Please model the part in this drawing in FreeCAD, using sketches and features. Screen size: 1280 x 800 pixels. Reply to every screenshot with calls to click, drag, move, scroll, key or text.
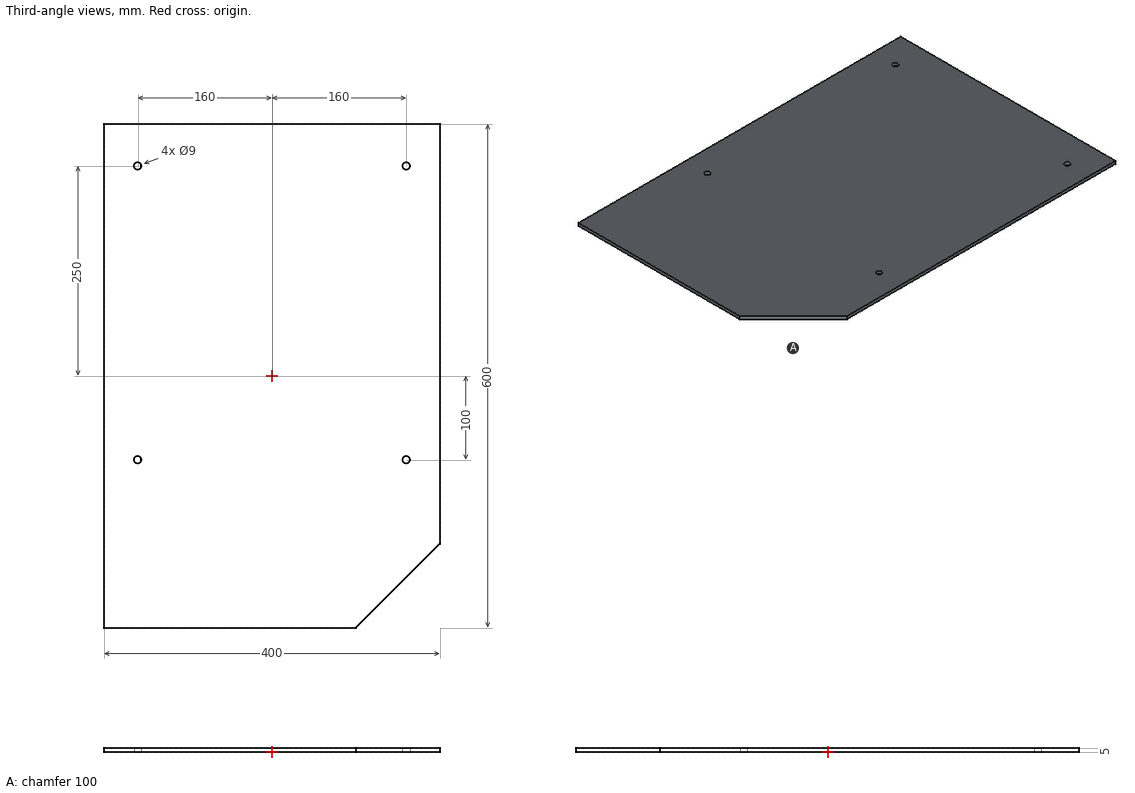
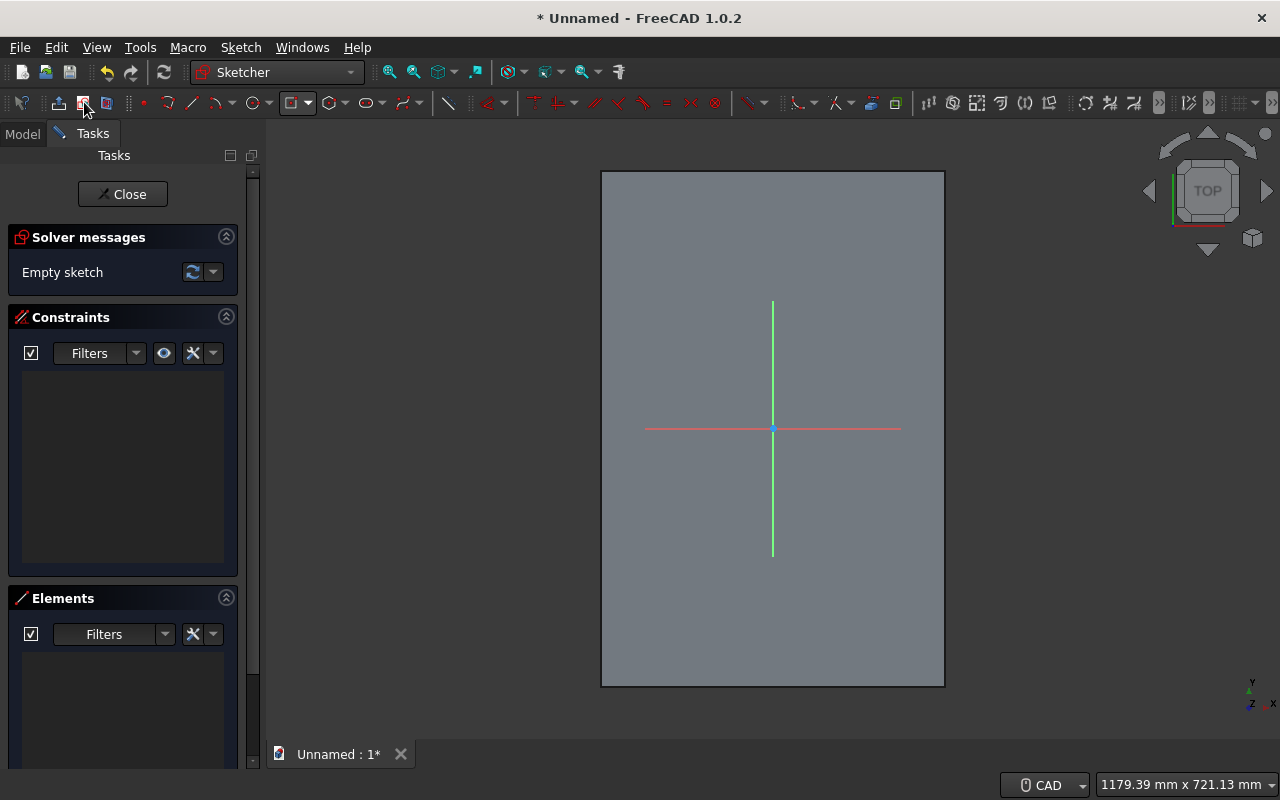
click(254, 104)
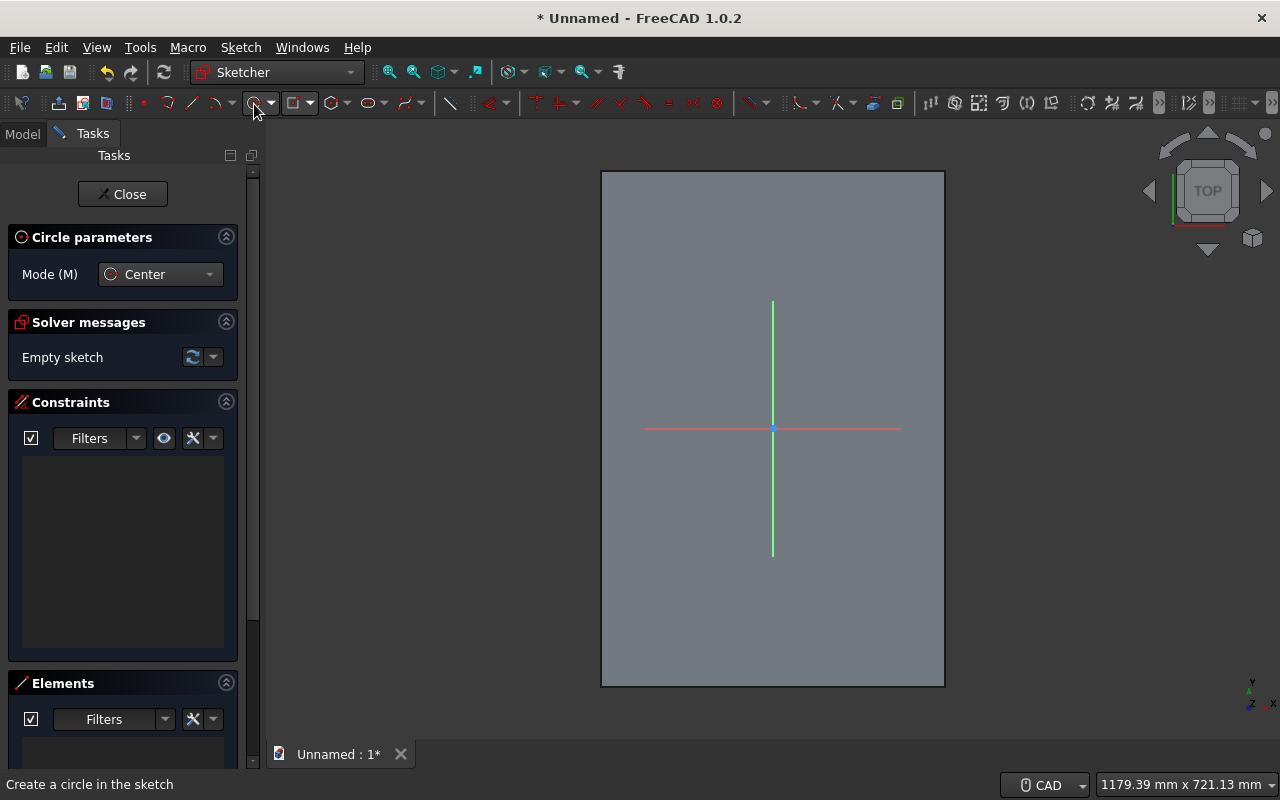
scroll(635, 214, up, 9)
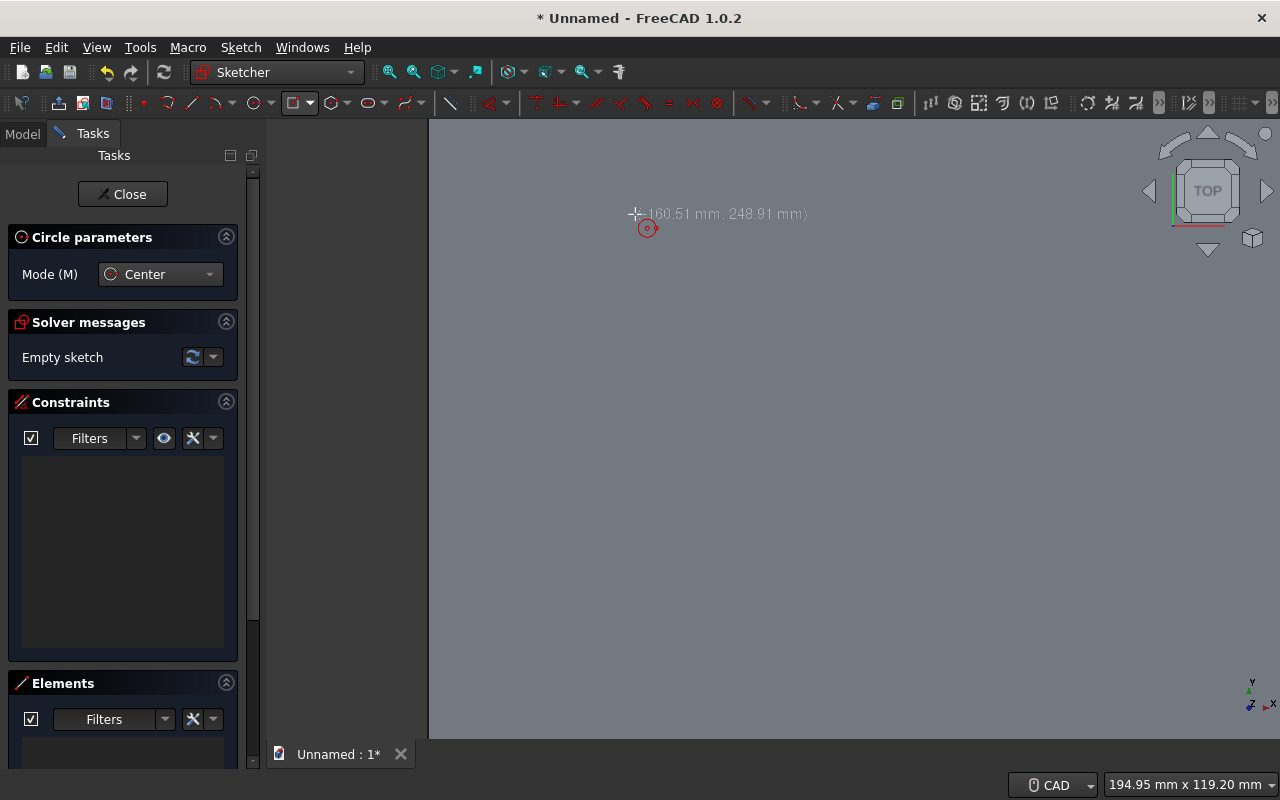
scroll(511, 253, down, 8)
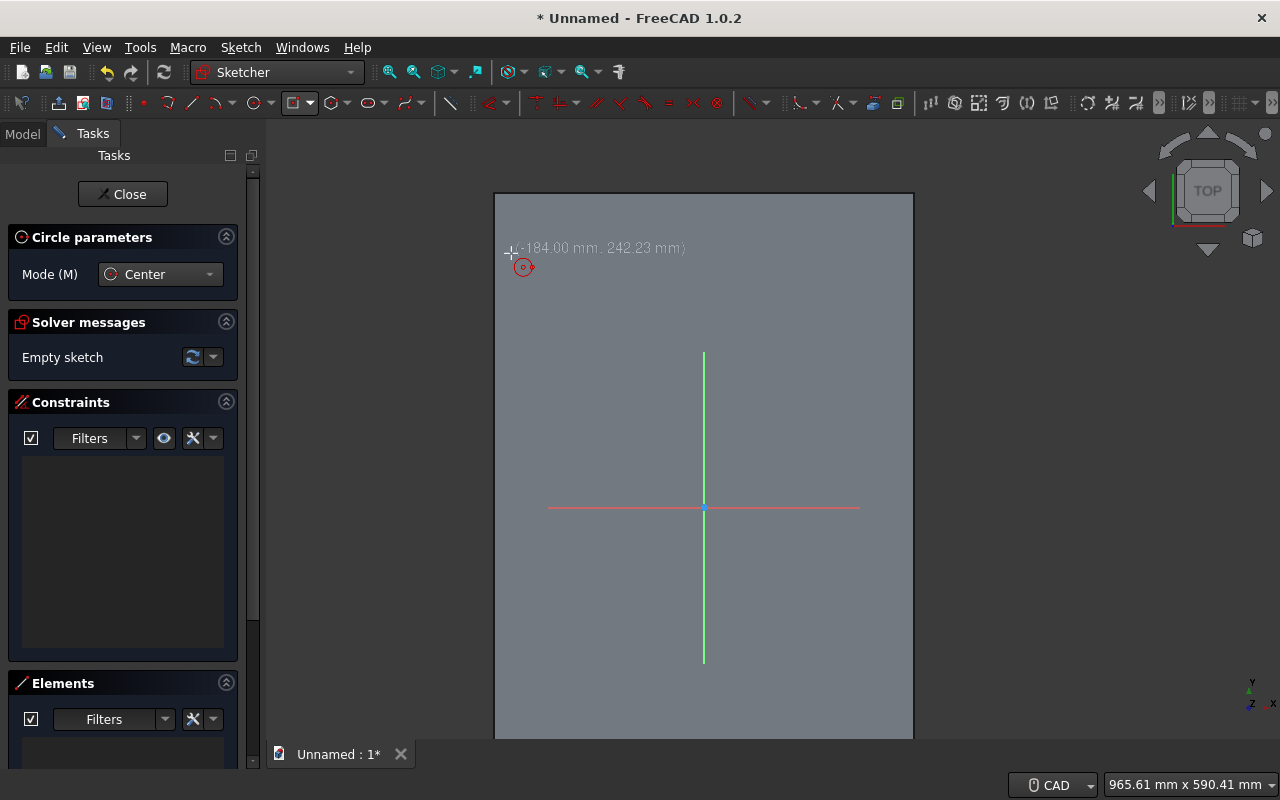
click(536, 245)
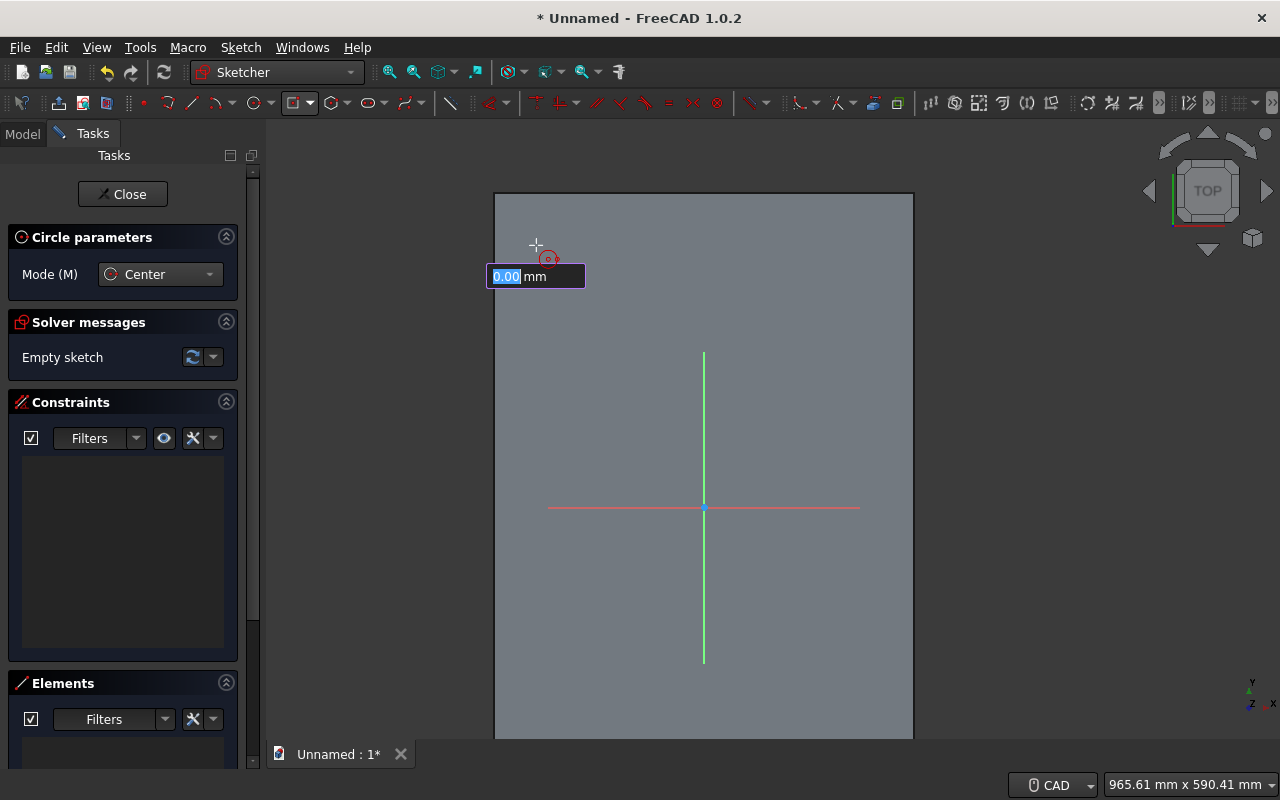
scroll(540, 242, up, 7)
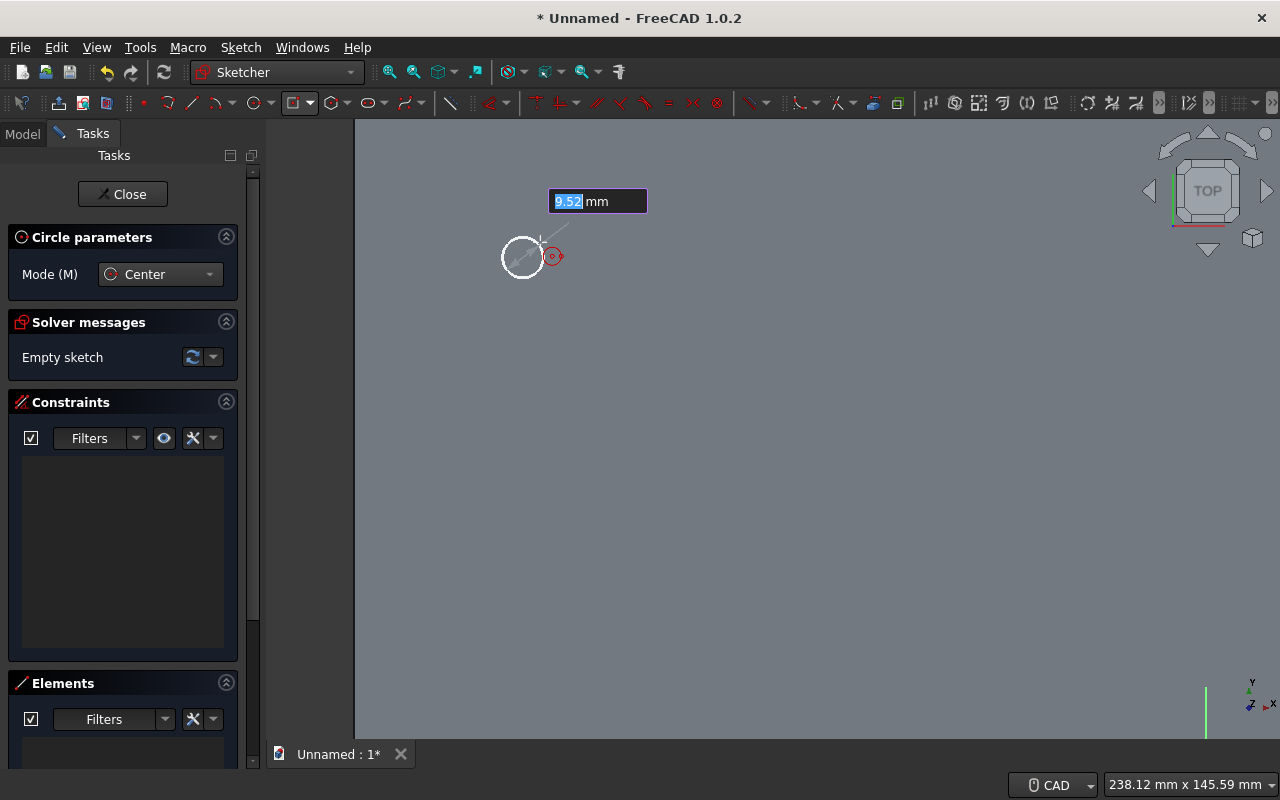
click(538, 241)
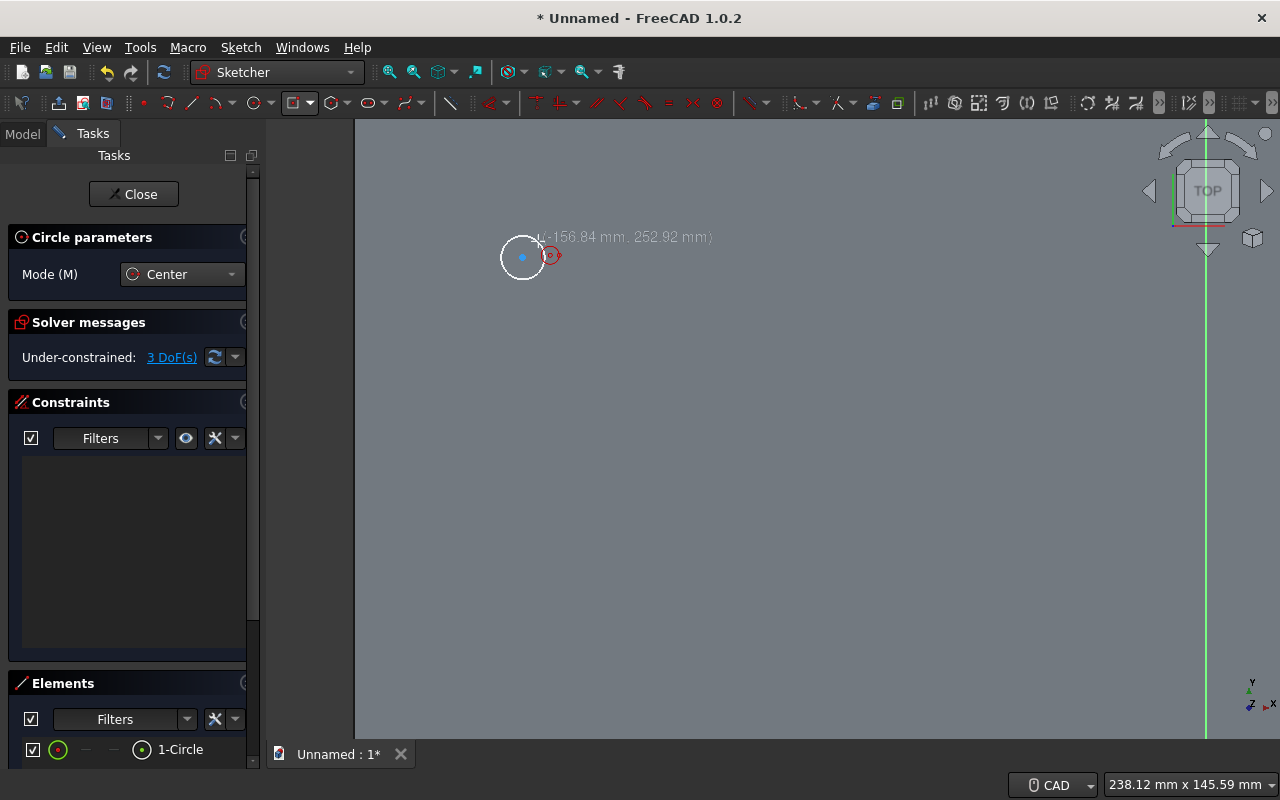
scroll(540, 242, down, 7)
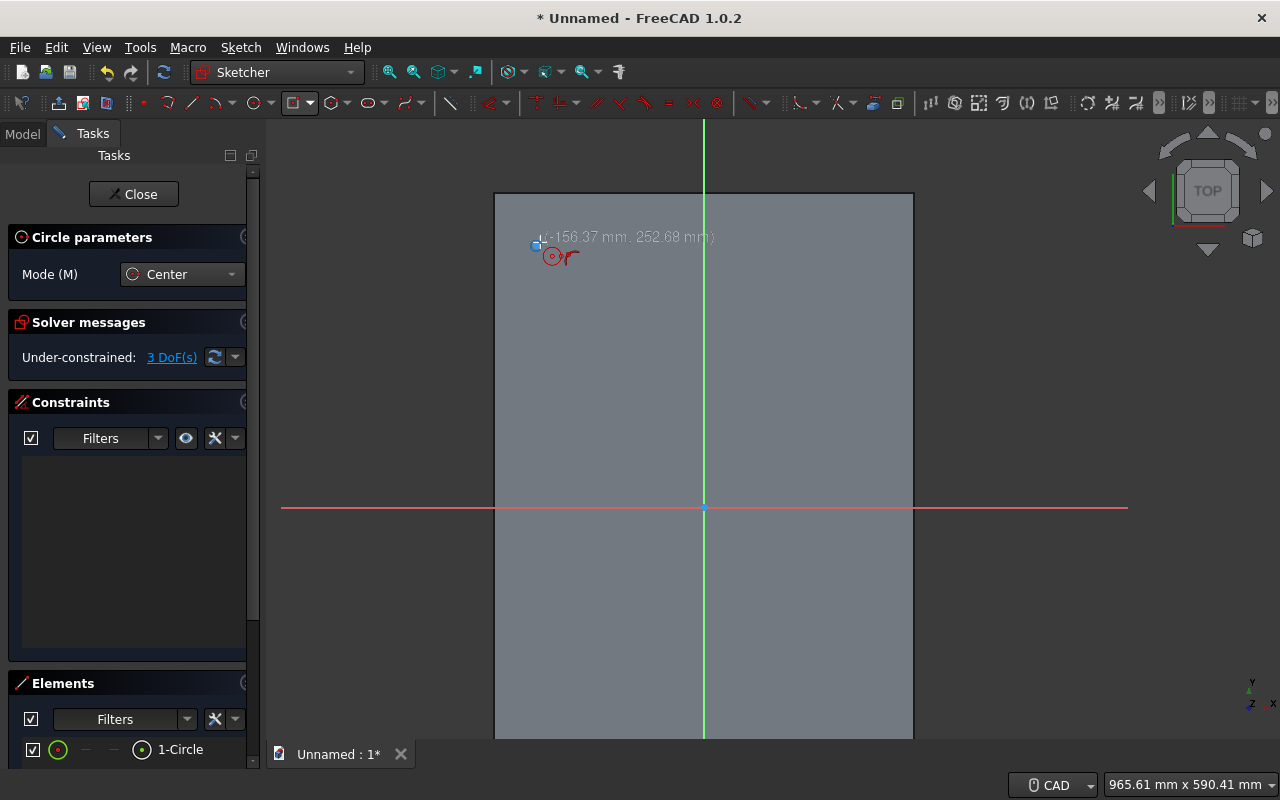
scroll(872, 245, up, 8)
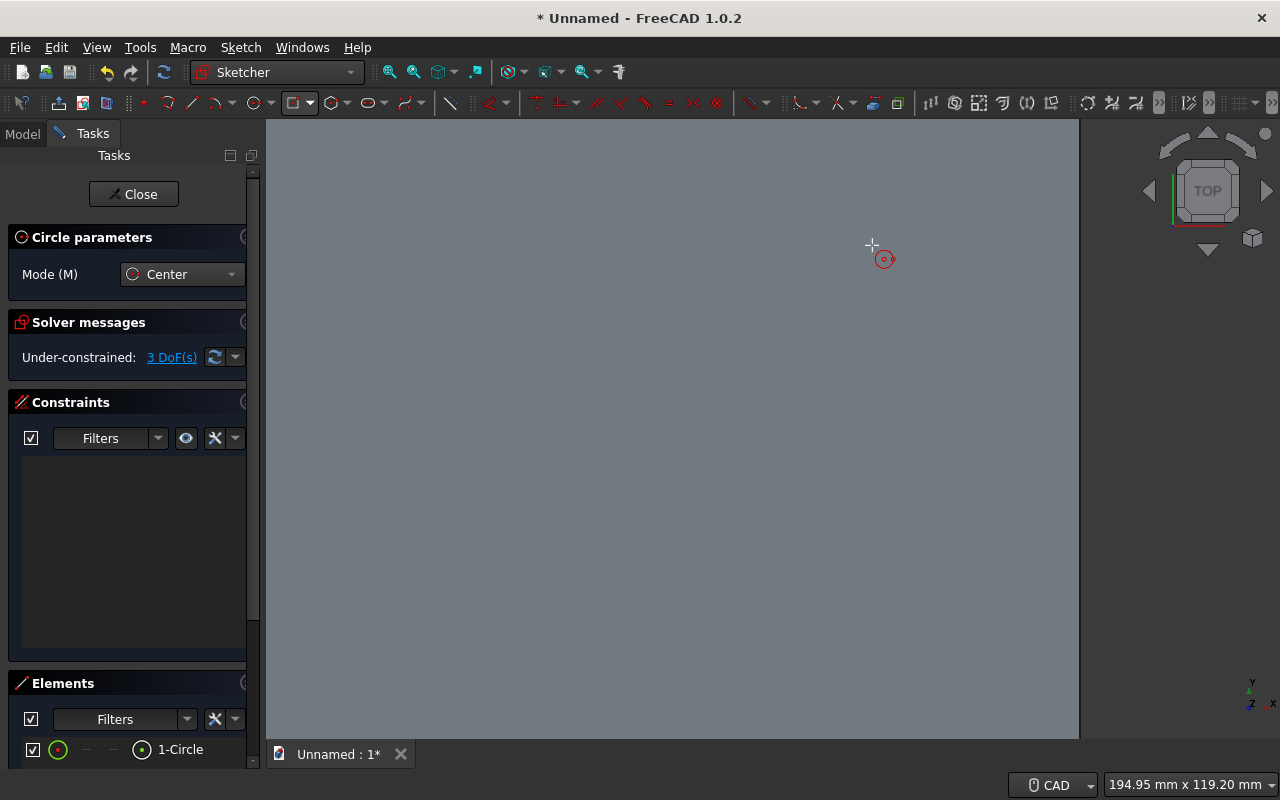
scroll(873, 245, down, 8)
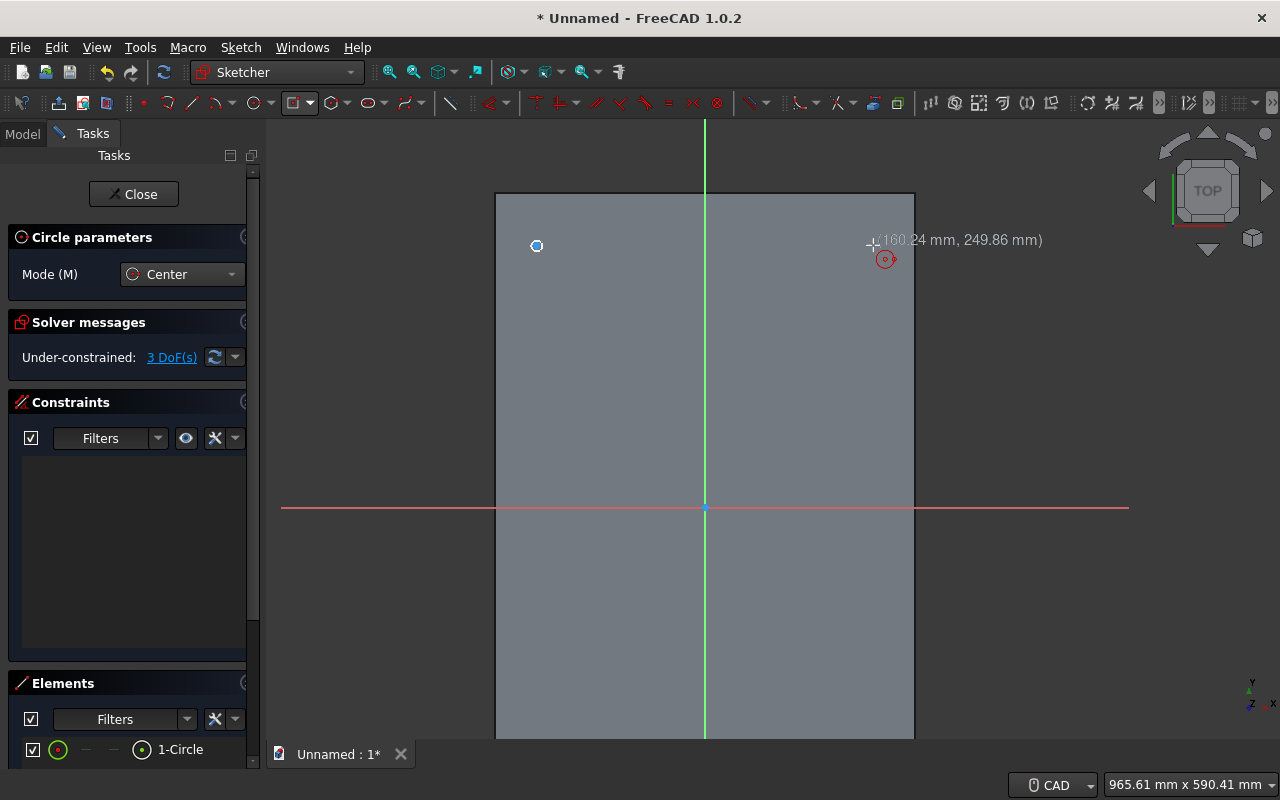
click(873, 245)